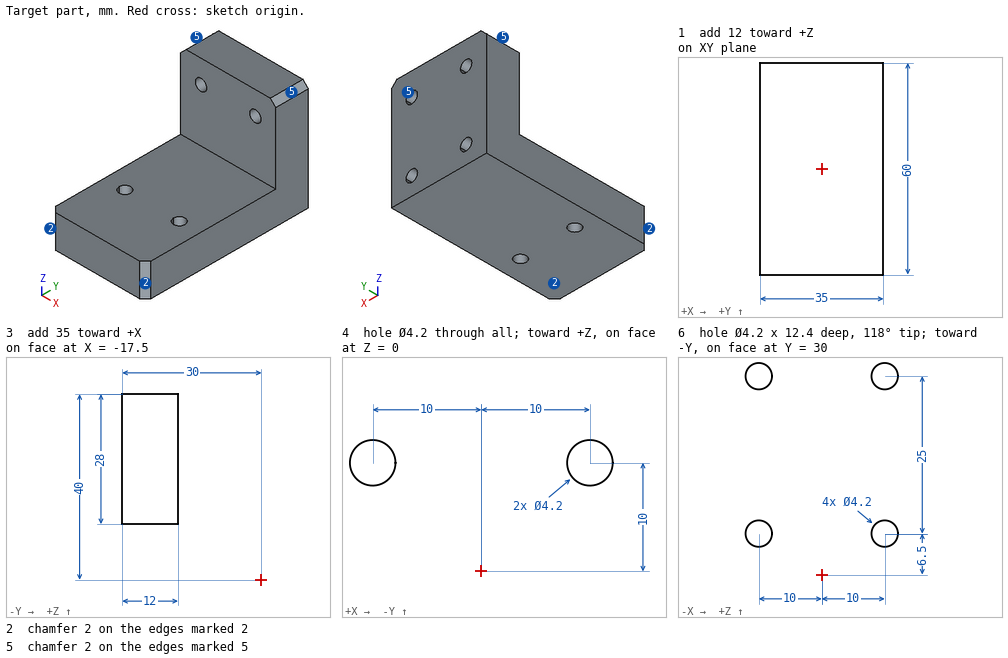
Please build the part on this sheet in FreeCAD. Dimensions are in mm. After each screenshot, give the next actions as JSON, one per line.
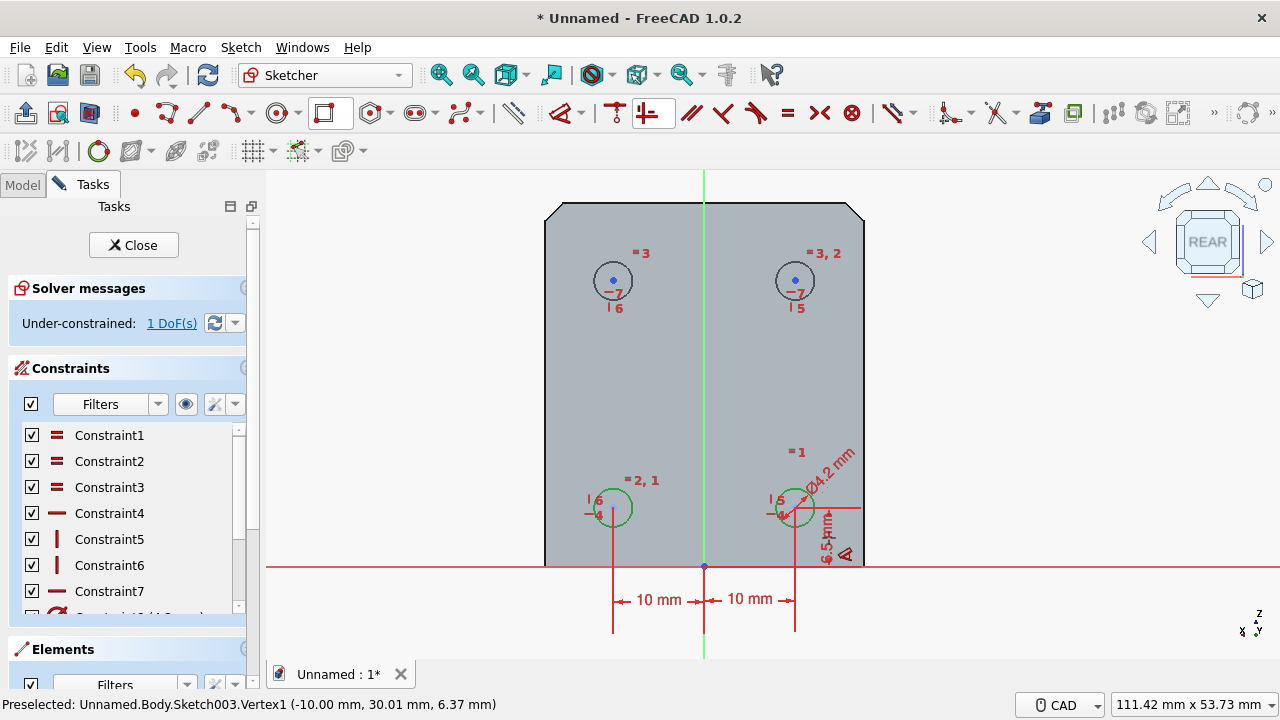
{"action": "left_click", "coordinate": [795, 508]}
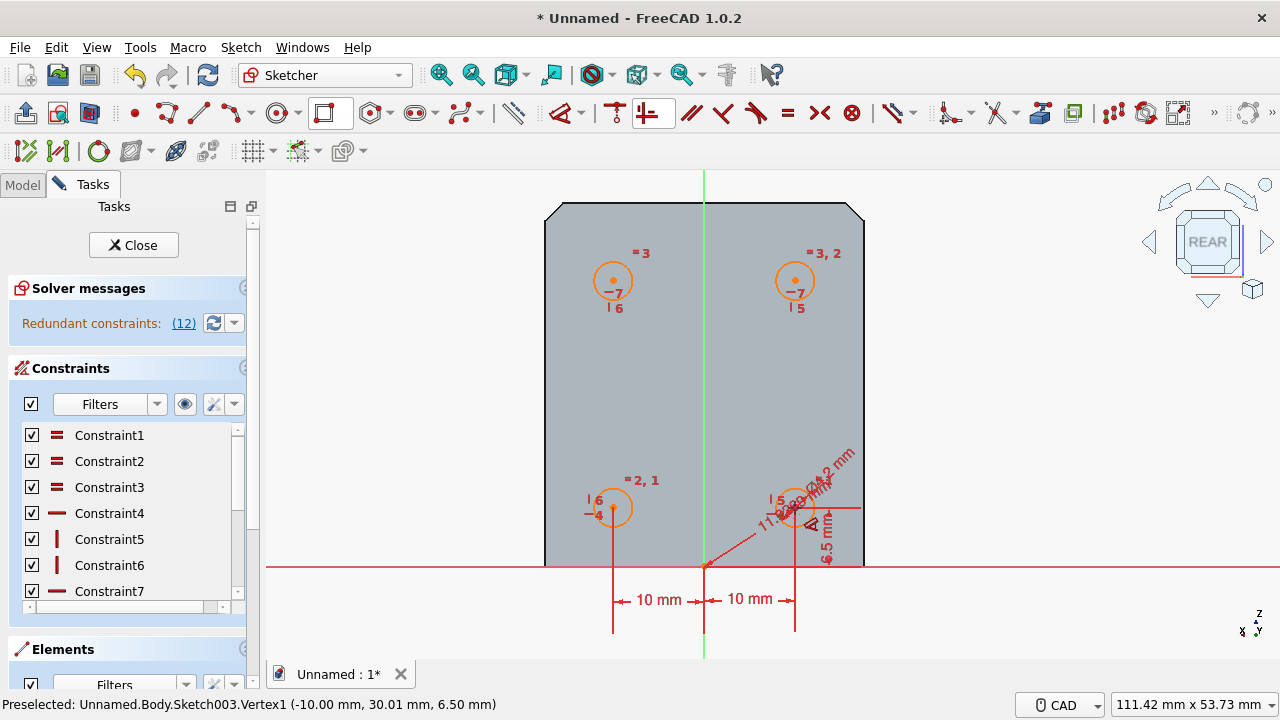
{"action": "left_click", "coordinate": [795, 281]}
{"action": "left_click", "coordinate": [829, 394]}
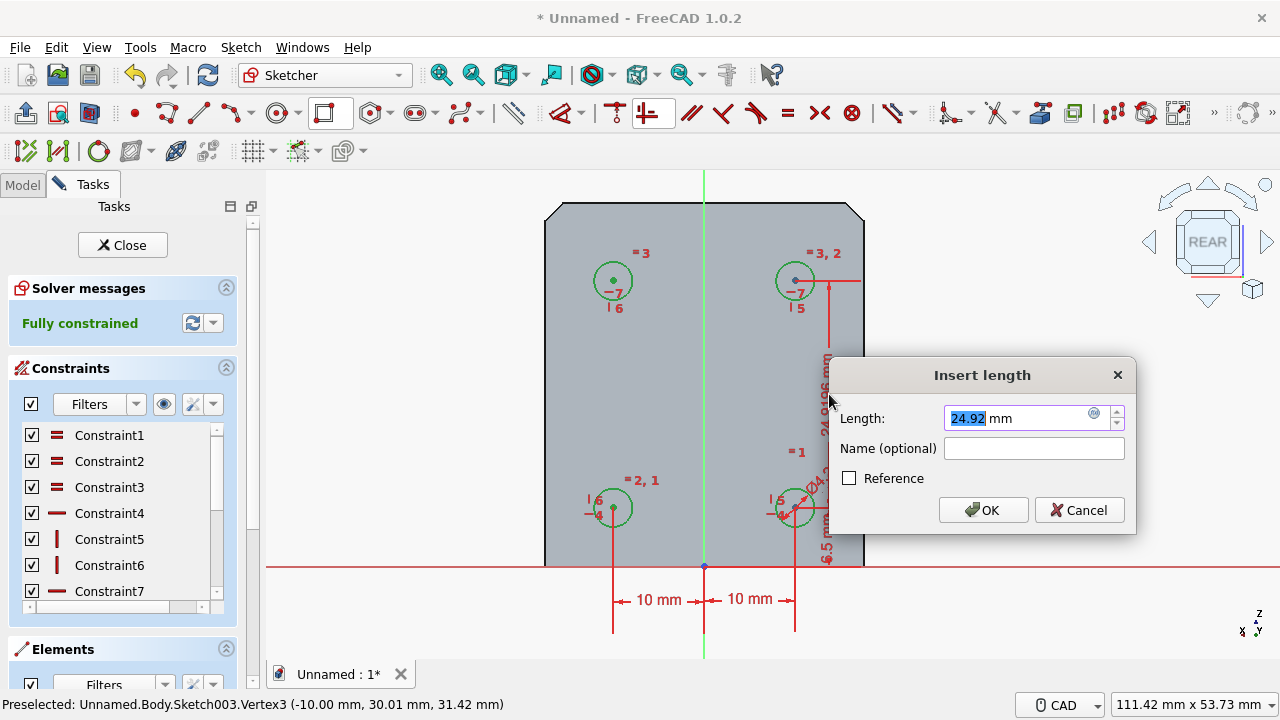
{"action": "type", "text": "25"}
{"action": "key", "text": "Return"}
{"action": "key", "text": "Escape"}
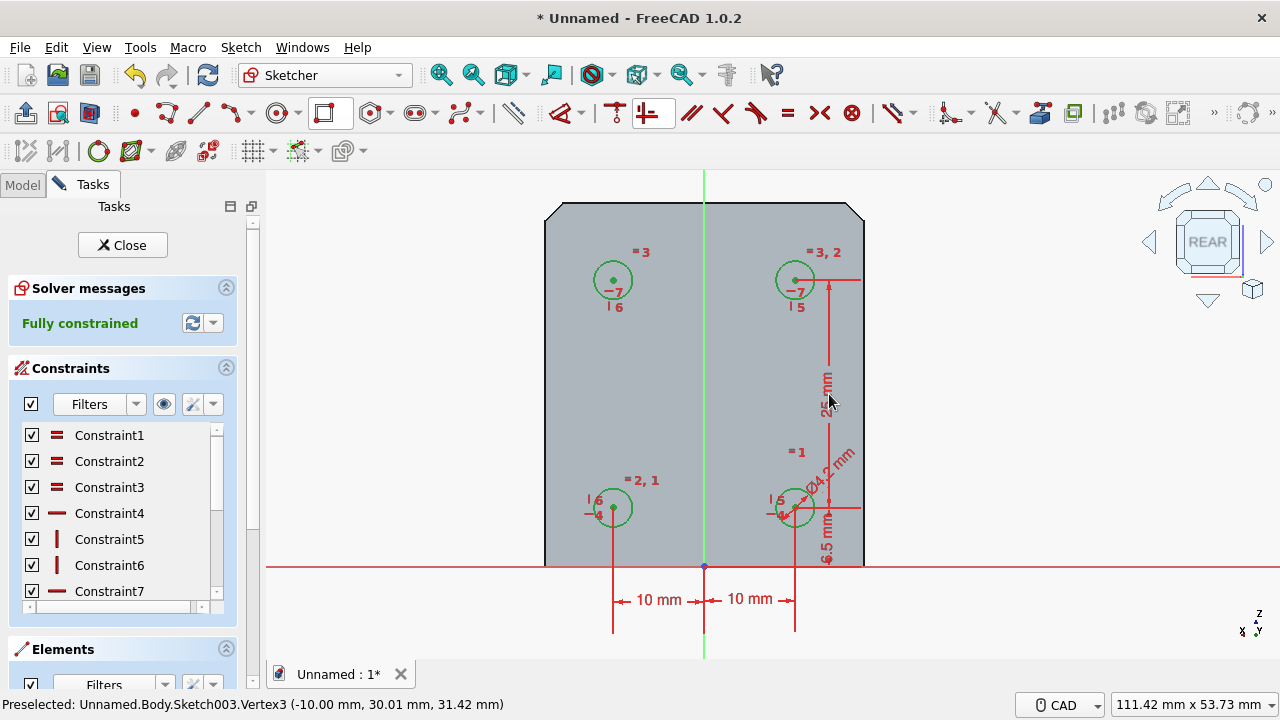
{"action": "left_click", "coordinate": [123, 245]}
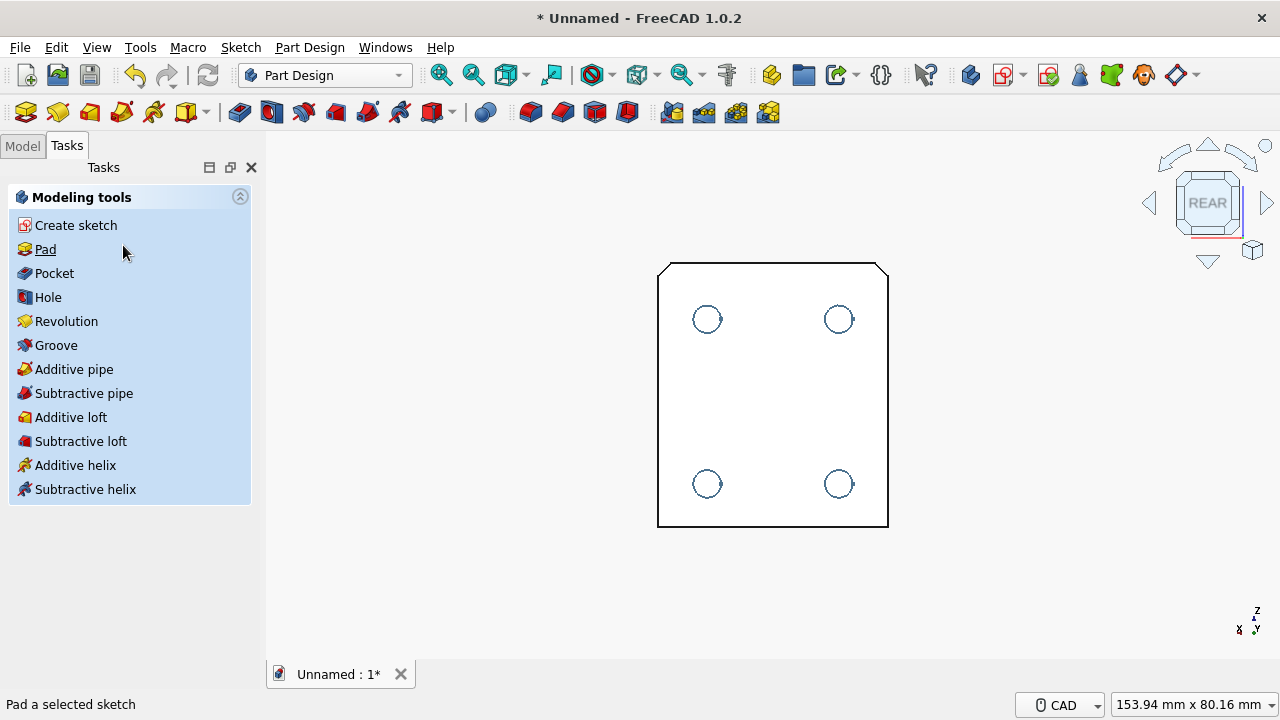
{"action": "left_click", "coordinate": [272, 112]}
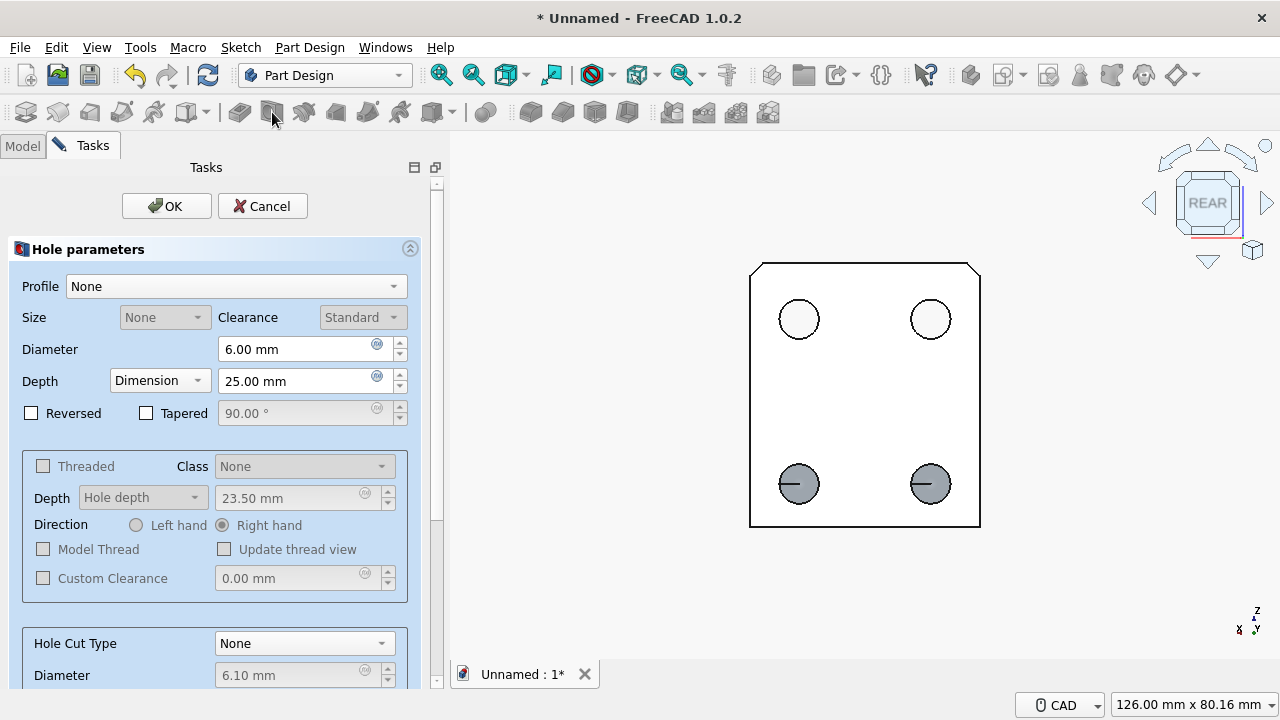
{"action": "triple_click", "coordinate": [305, 349]}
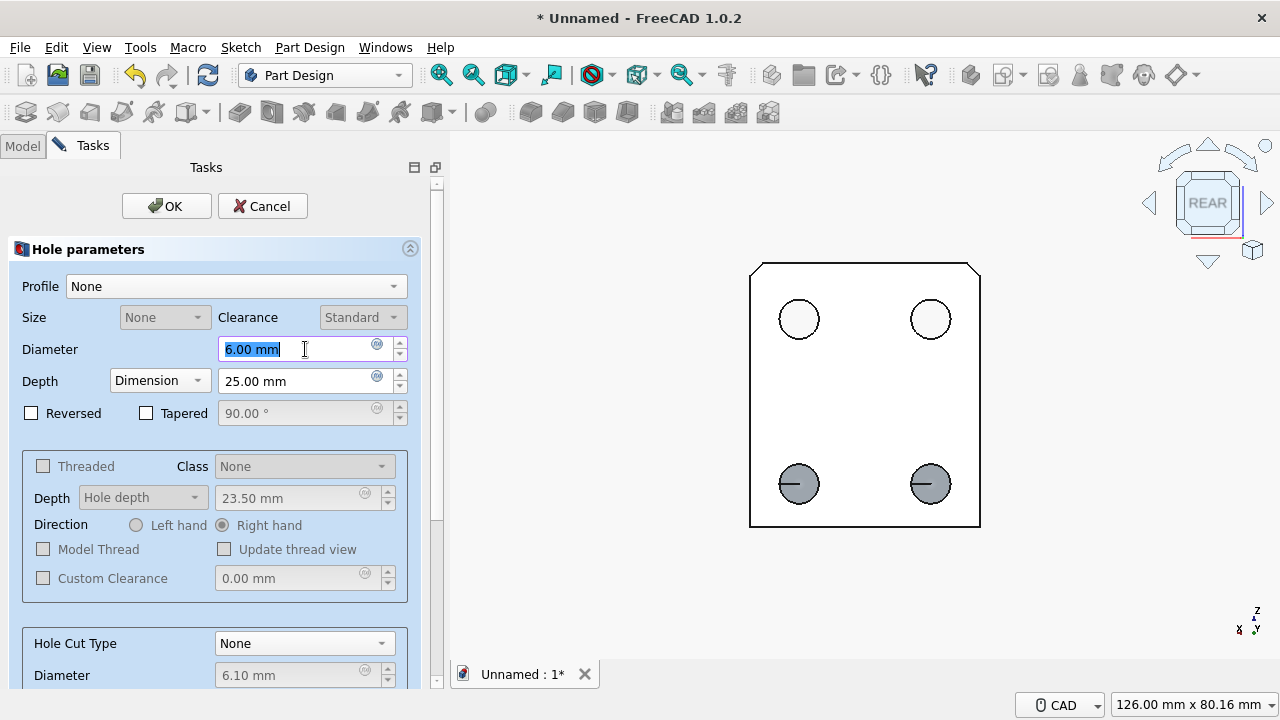
{"action": "type", "text": "4.2"}
{"action": "key", "text": "Tab"}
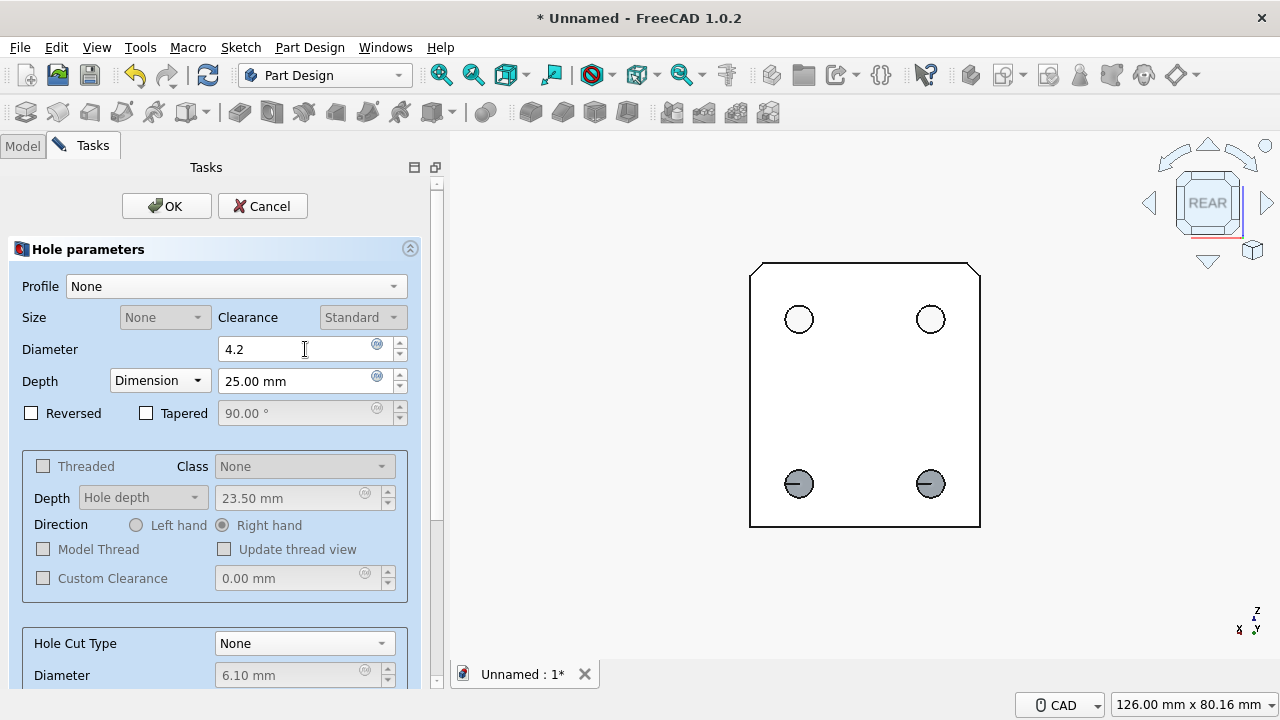
{"action": "triple_click", "coordinate": [305, 381]}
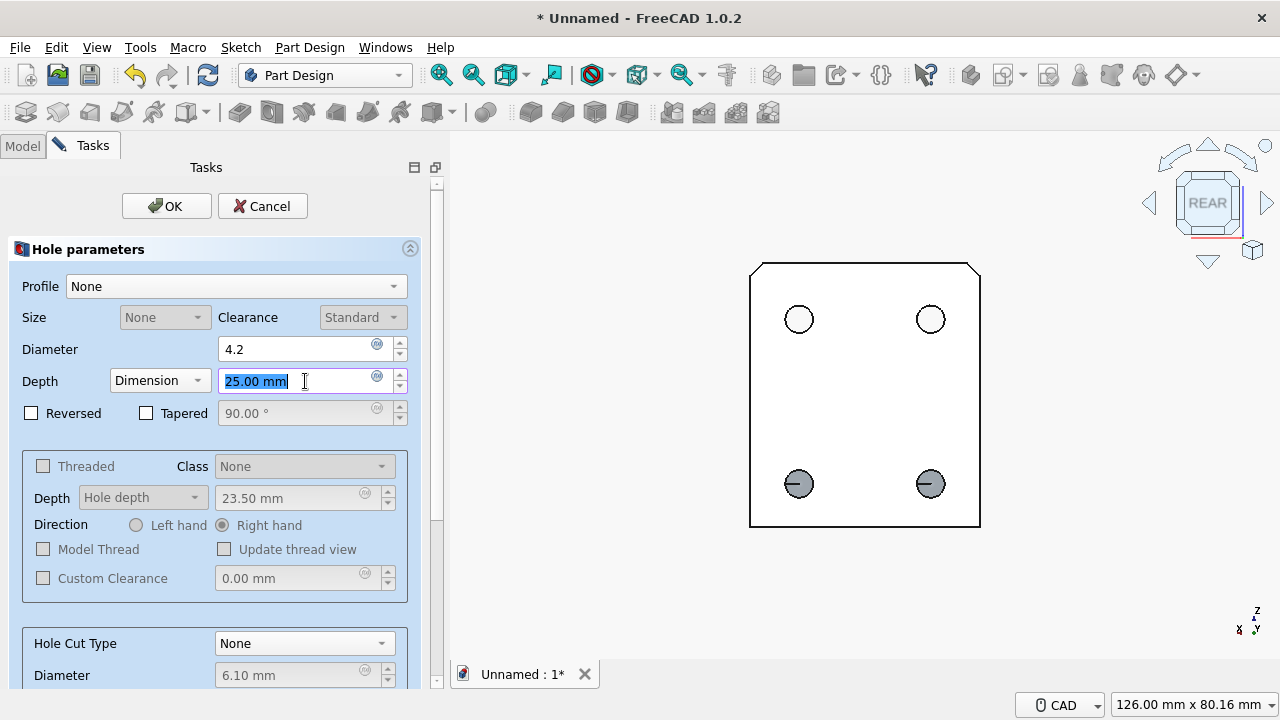
{"action": "type", "text": "12.4"}
{"action": "key", "text": "Tab"}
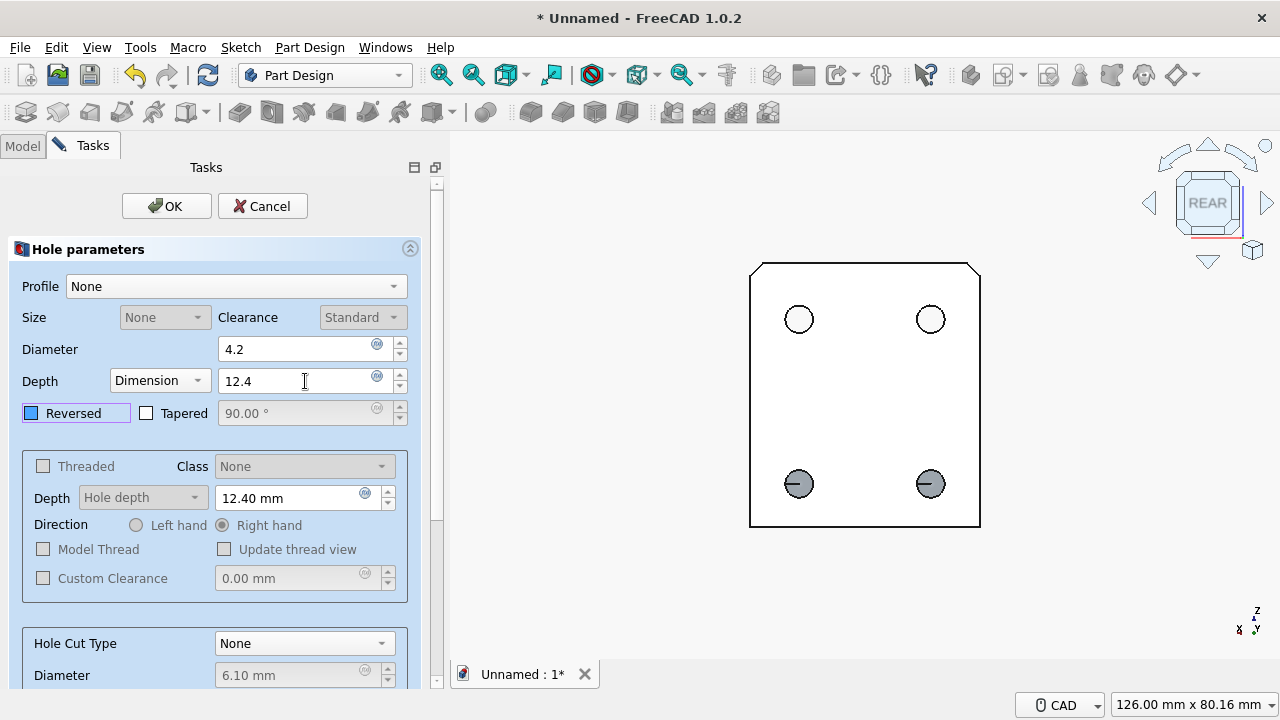
{"action": "left_click", "coordinate": [167, 206]}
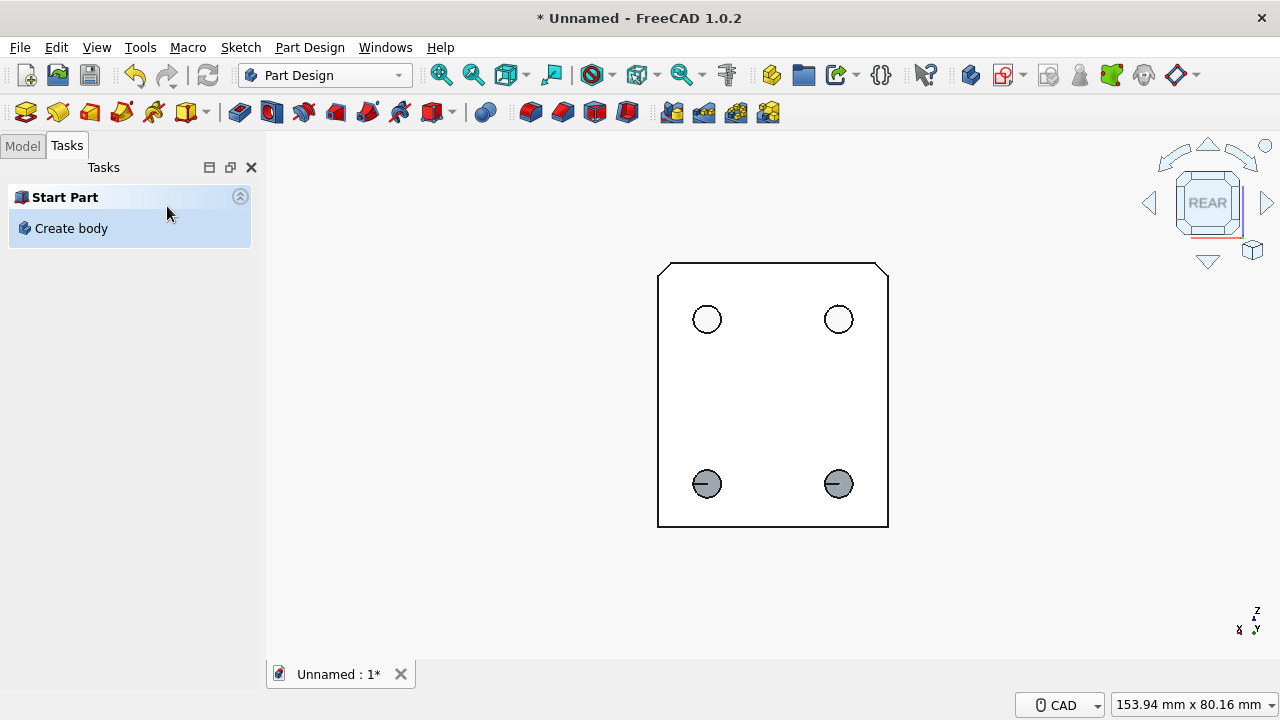
{"action": "key", "text": "0"}